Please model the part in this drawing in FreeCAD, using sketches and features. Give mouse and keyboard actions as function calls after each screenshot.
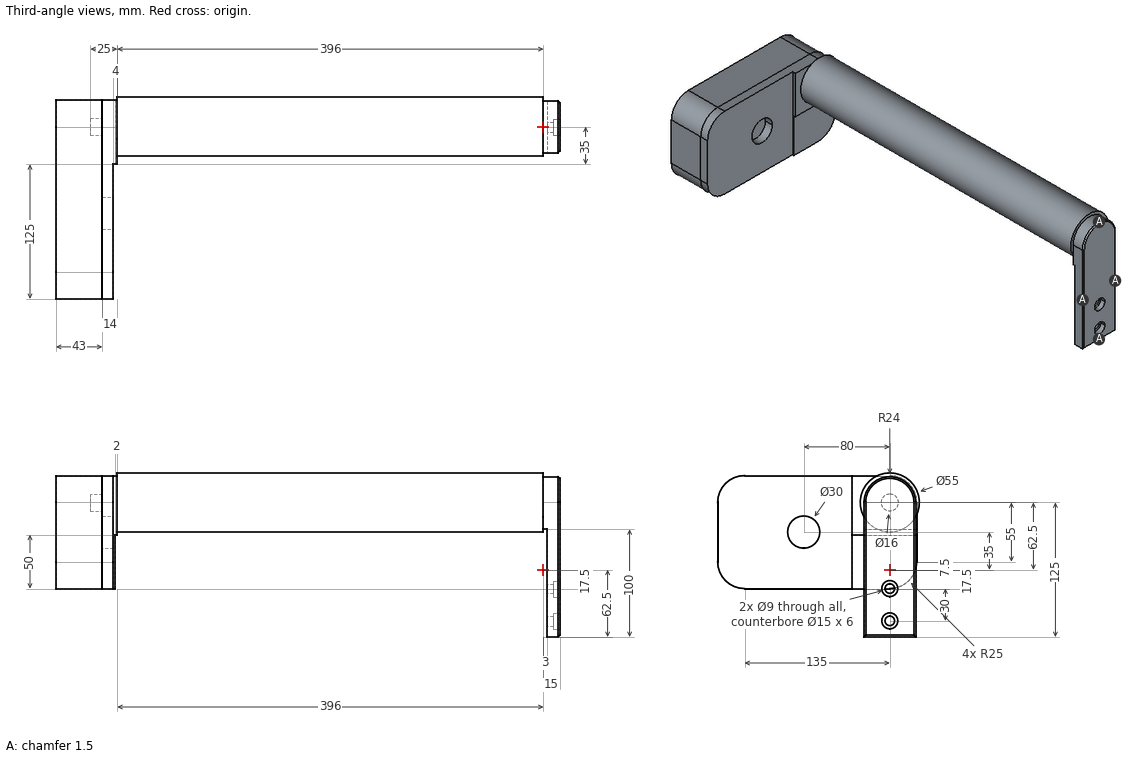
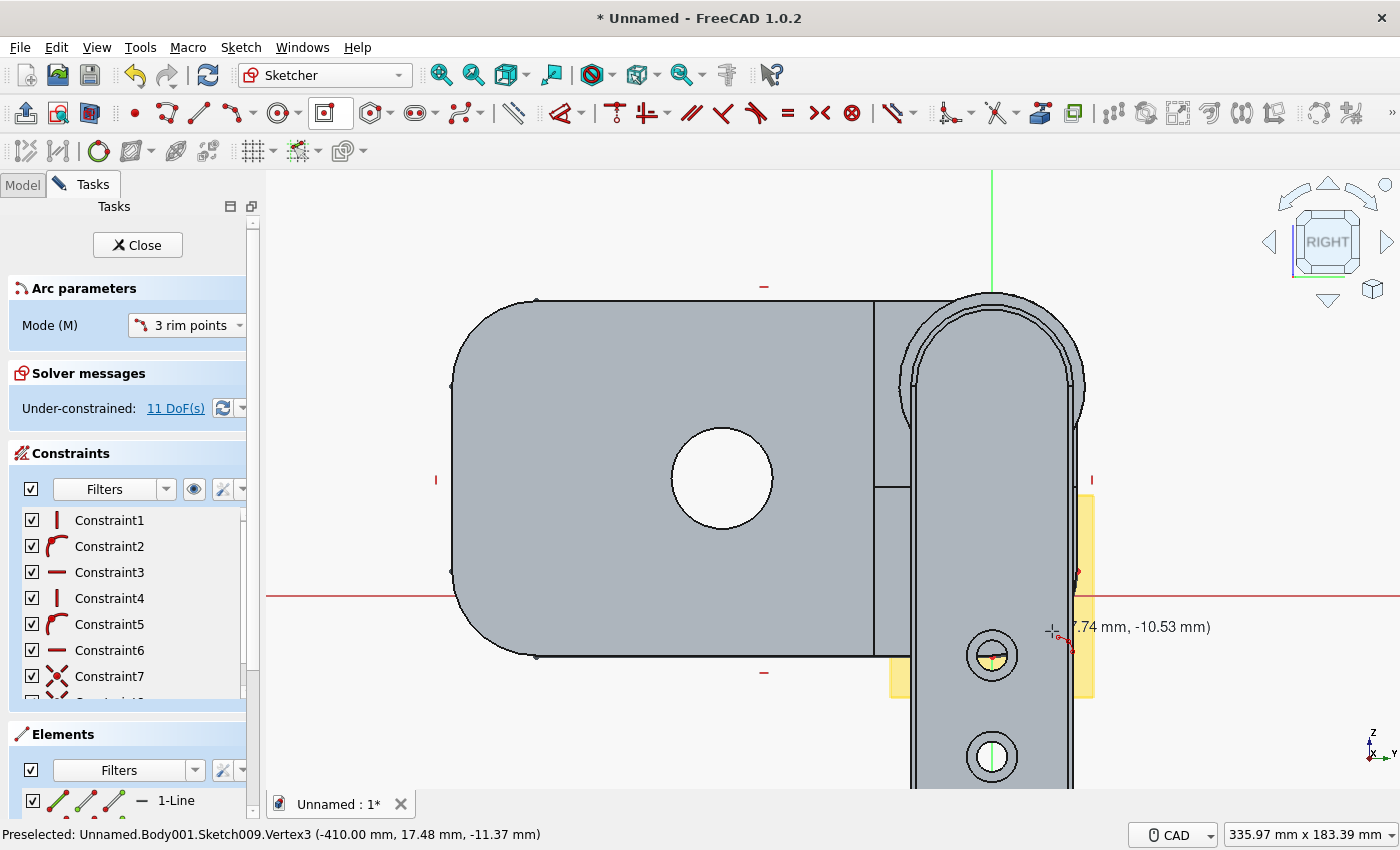
click(536, 657)
click(452, 572)
click(477, 631)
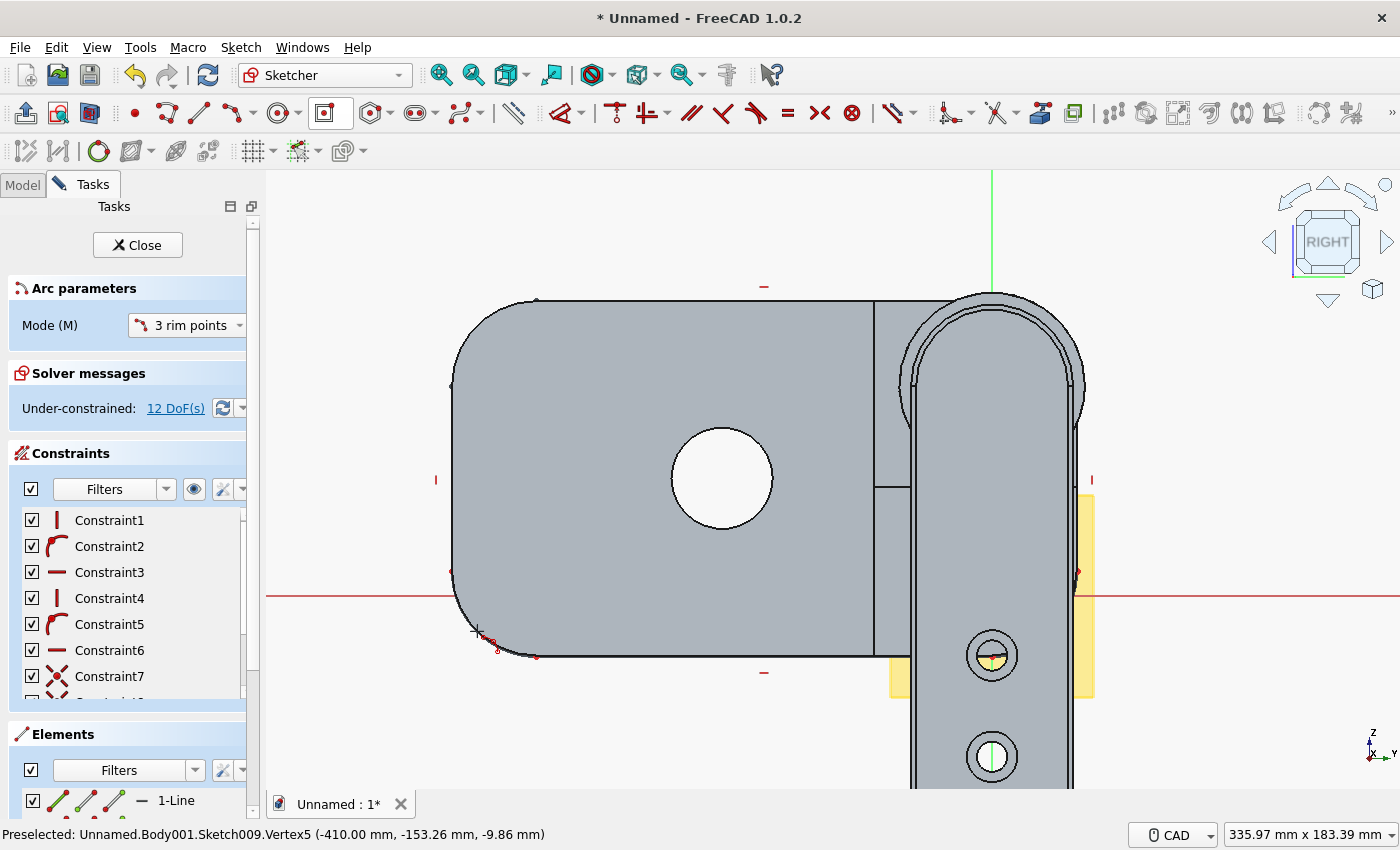
click(452, 387)
click(536, 302)
click(477, 326)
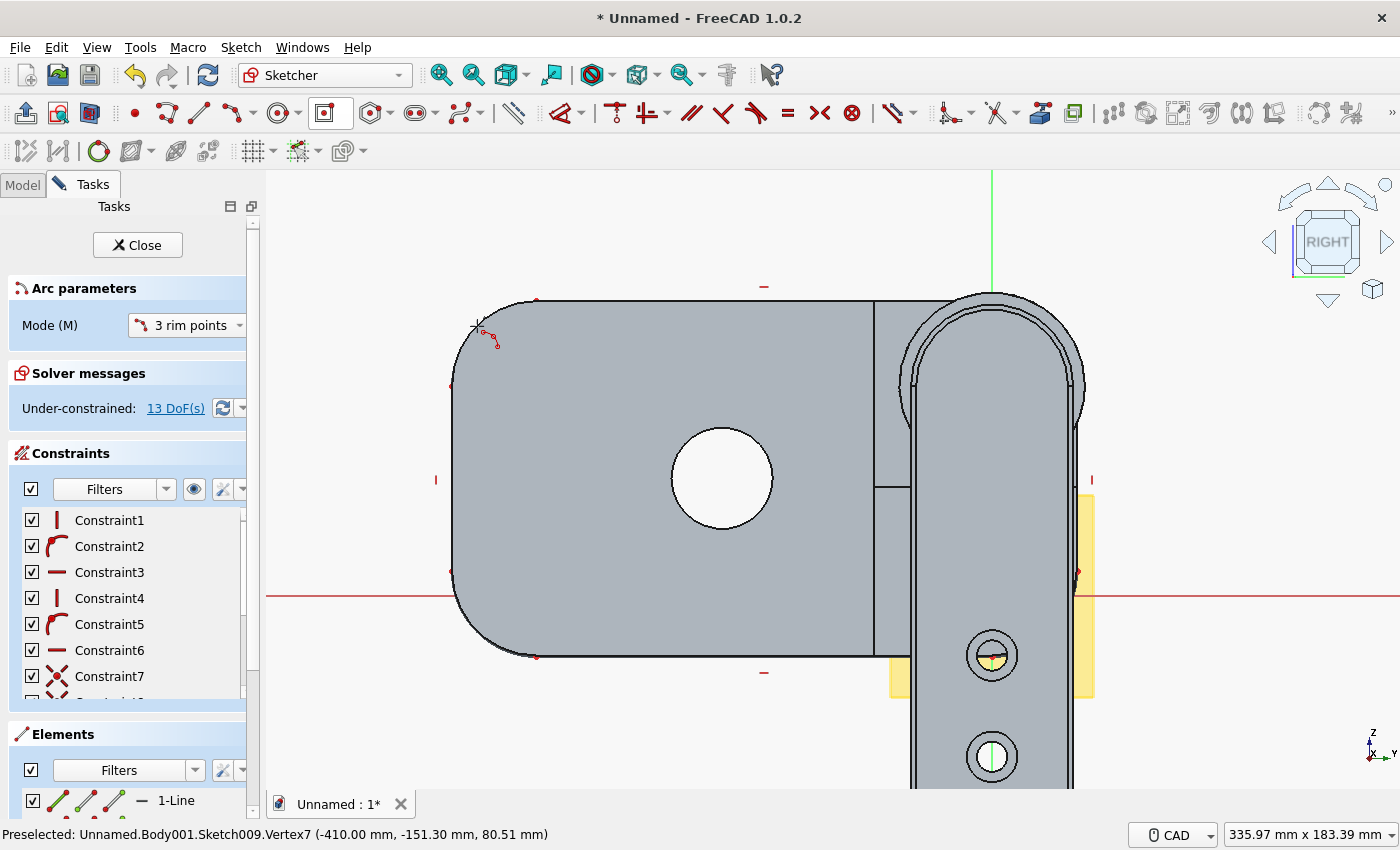
click(992, 302)
click(1077, 387)
click(1052, 326)
key(Escape)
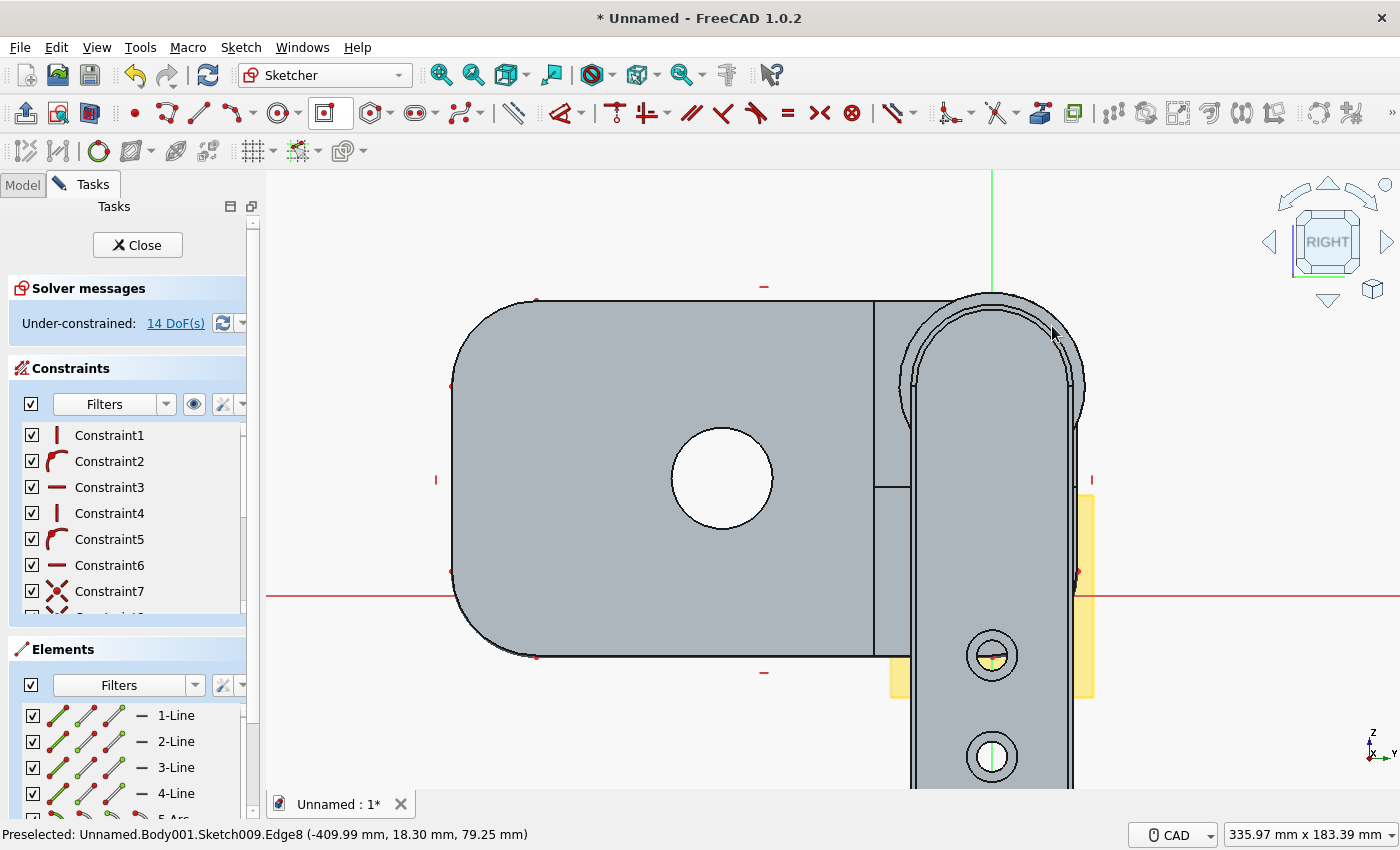
click(1077, 443)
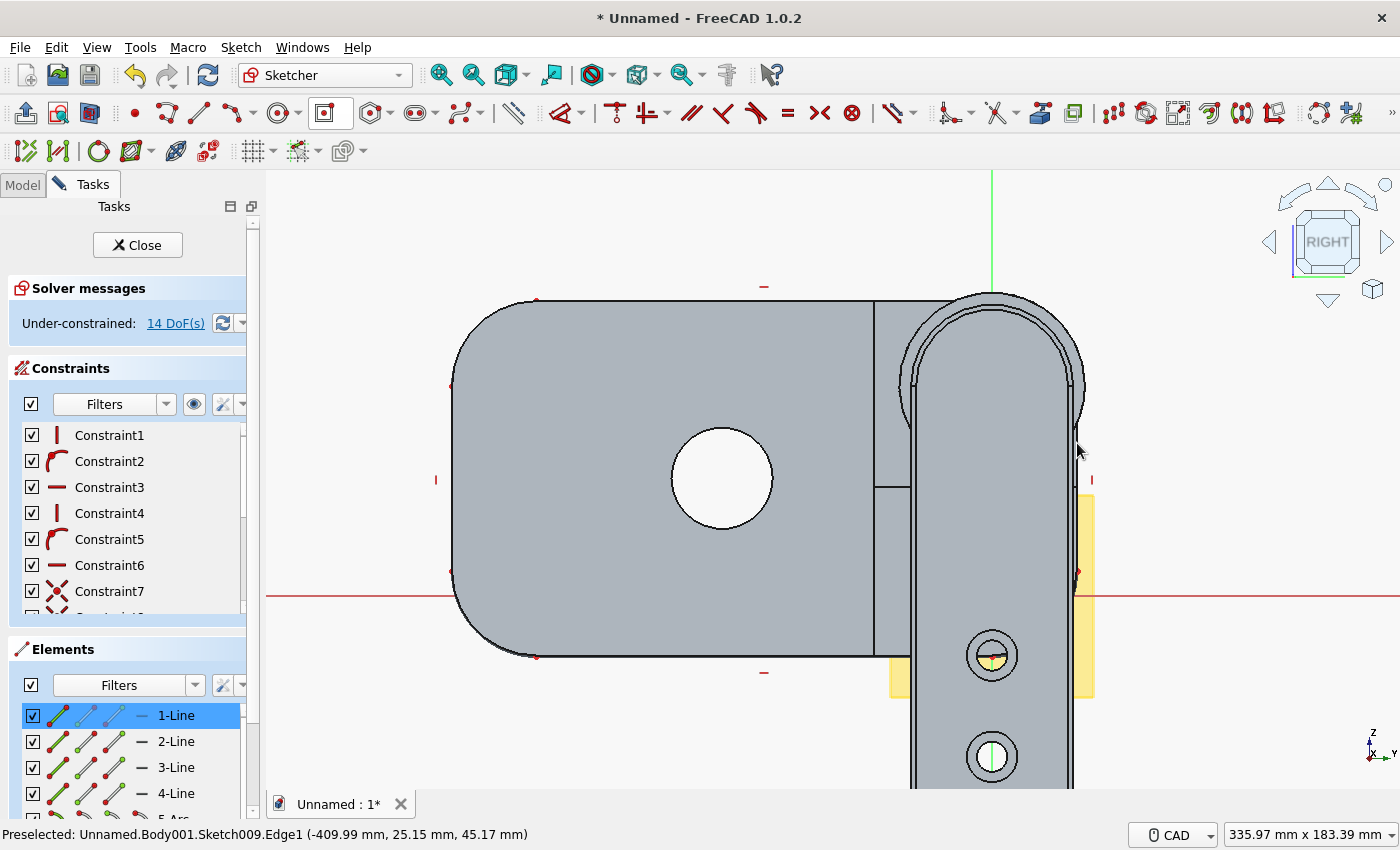
click(1031, 648)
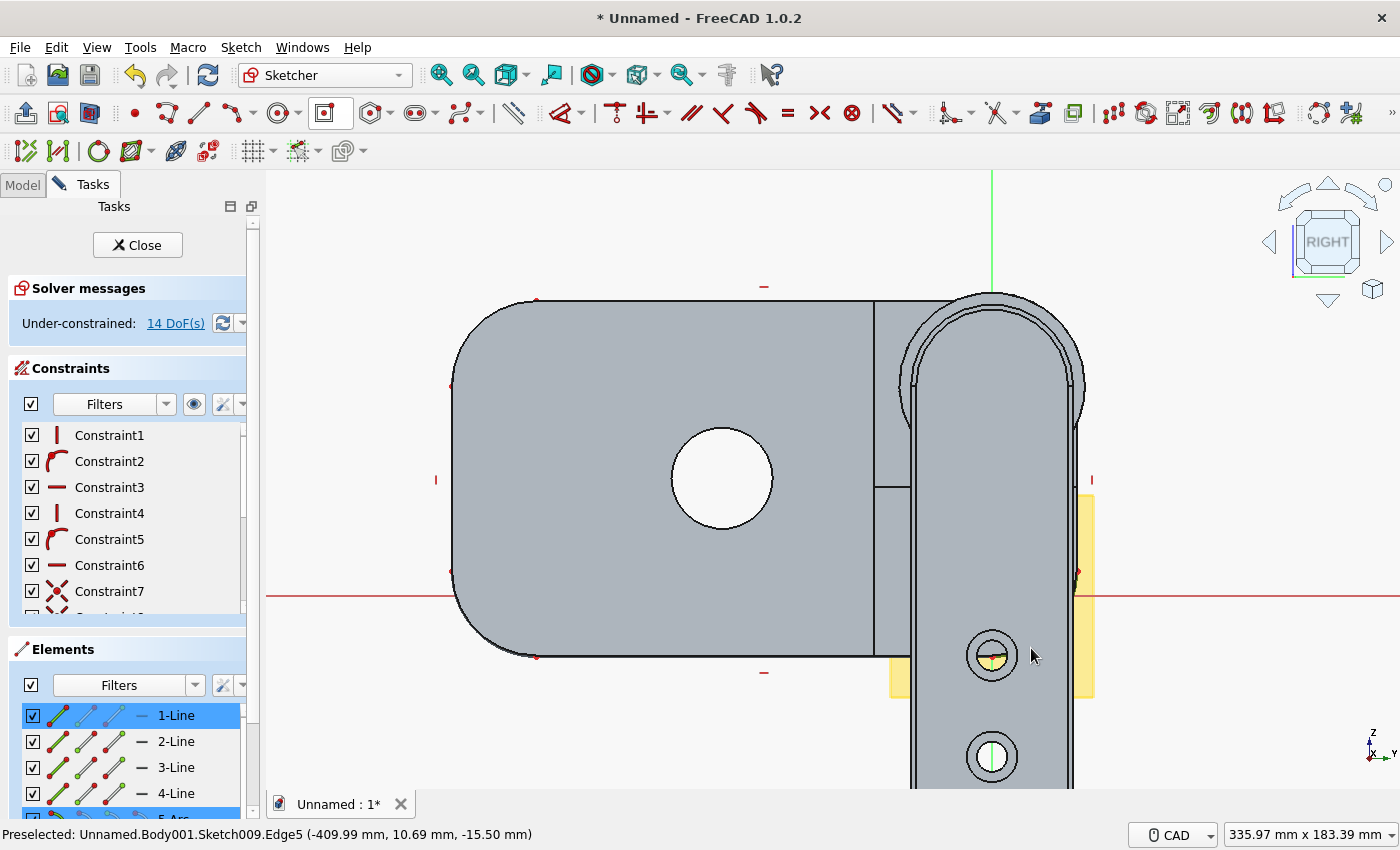
key(t)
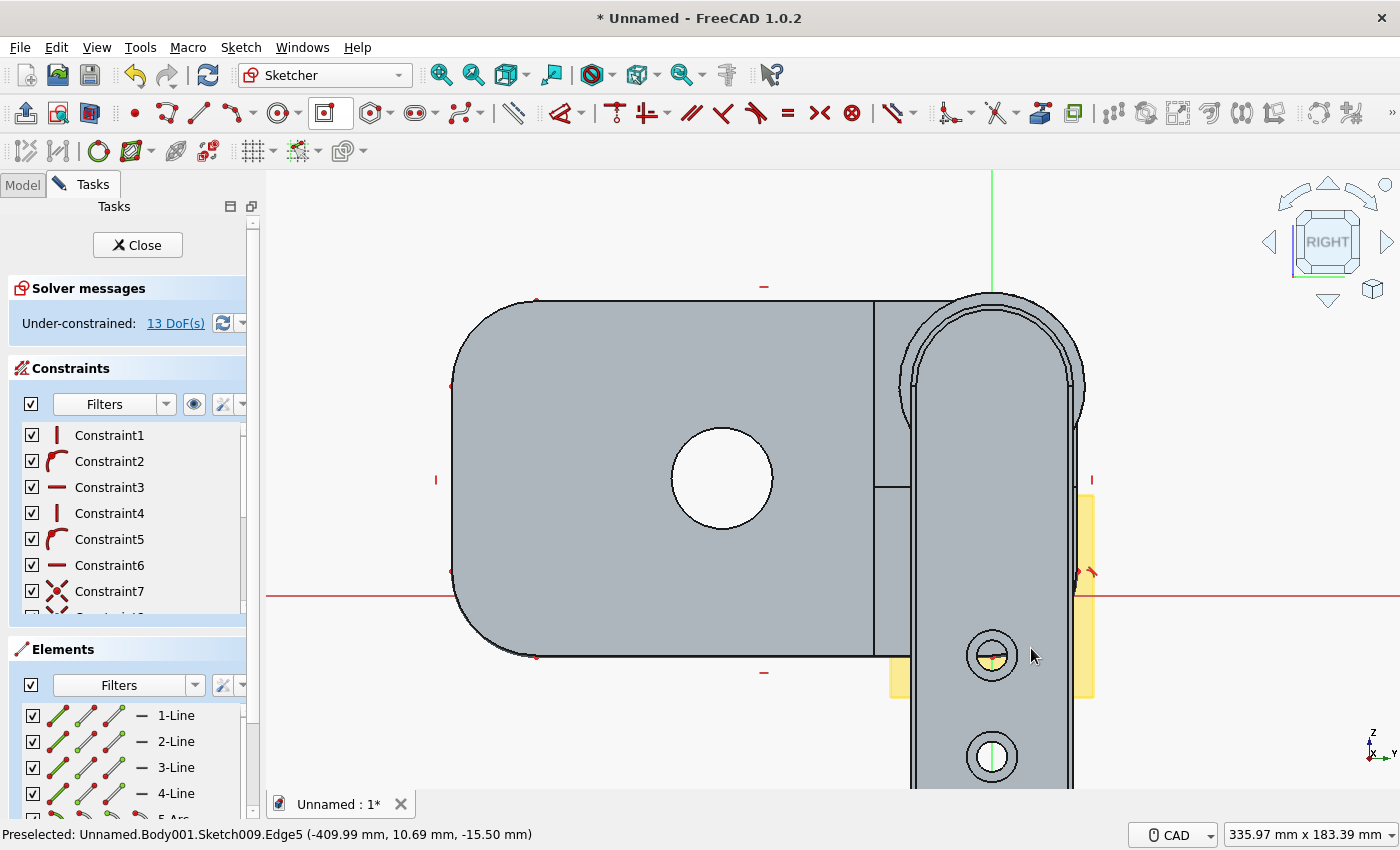
click(1077, 442)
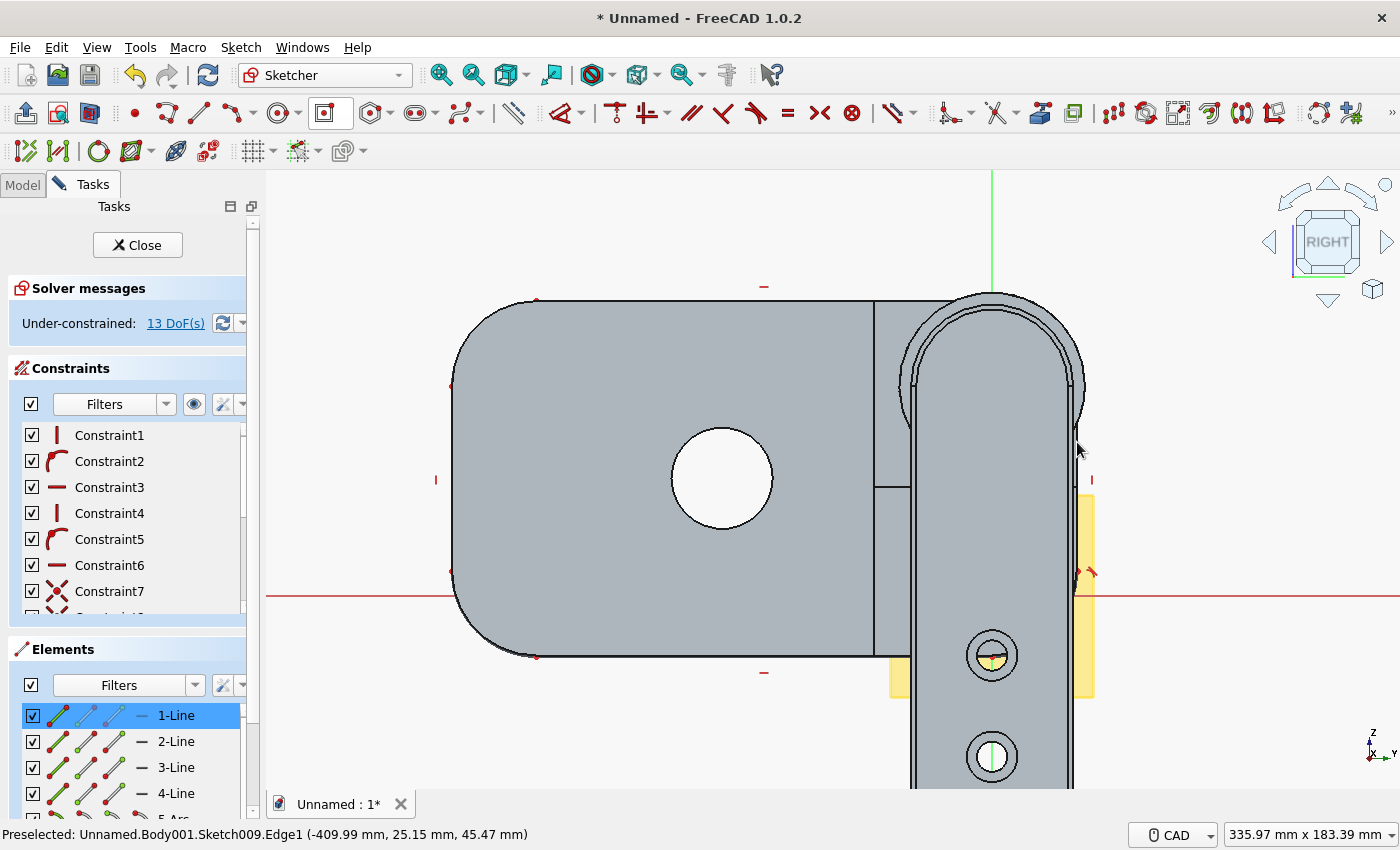
click(1068, 349)